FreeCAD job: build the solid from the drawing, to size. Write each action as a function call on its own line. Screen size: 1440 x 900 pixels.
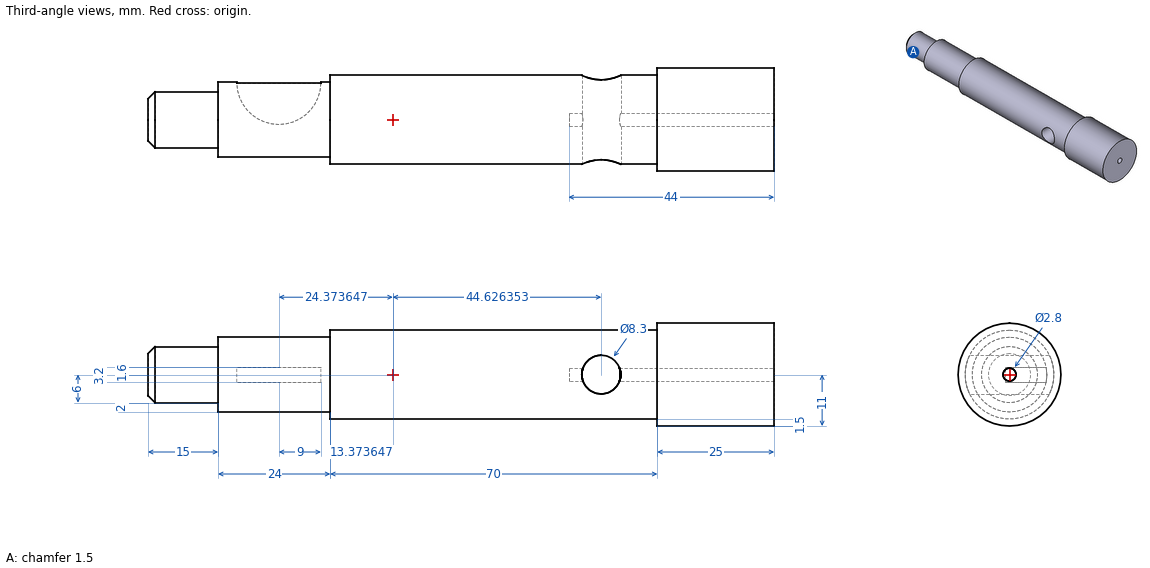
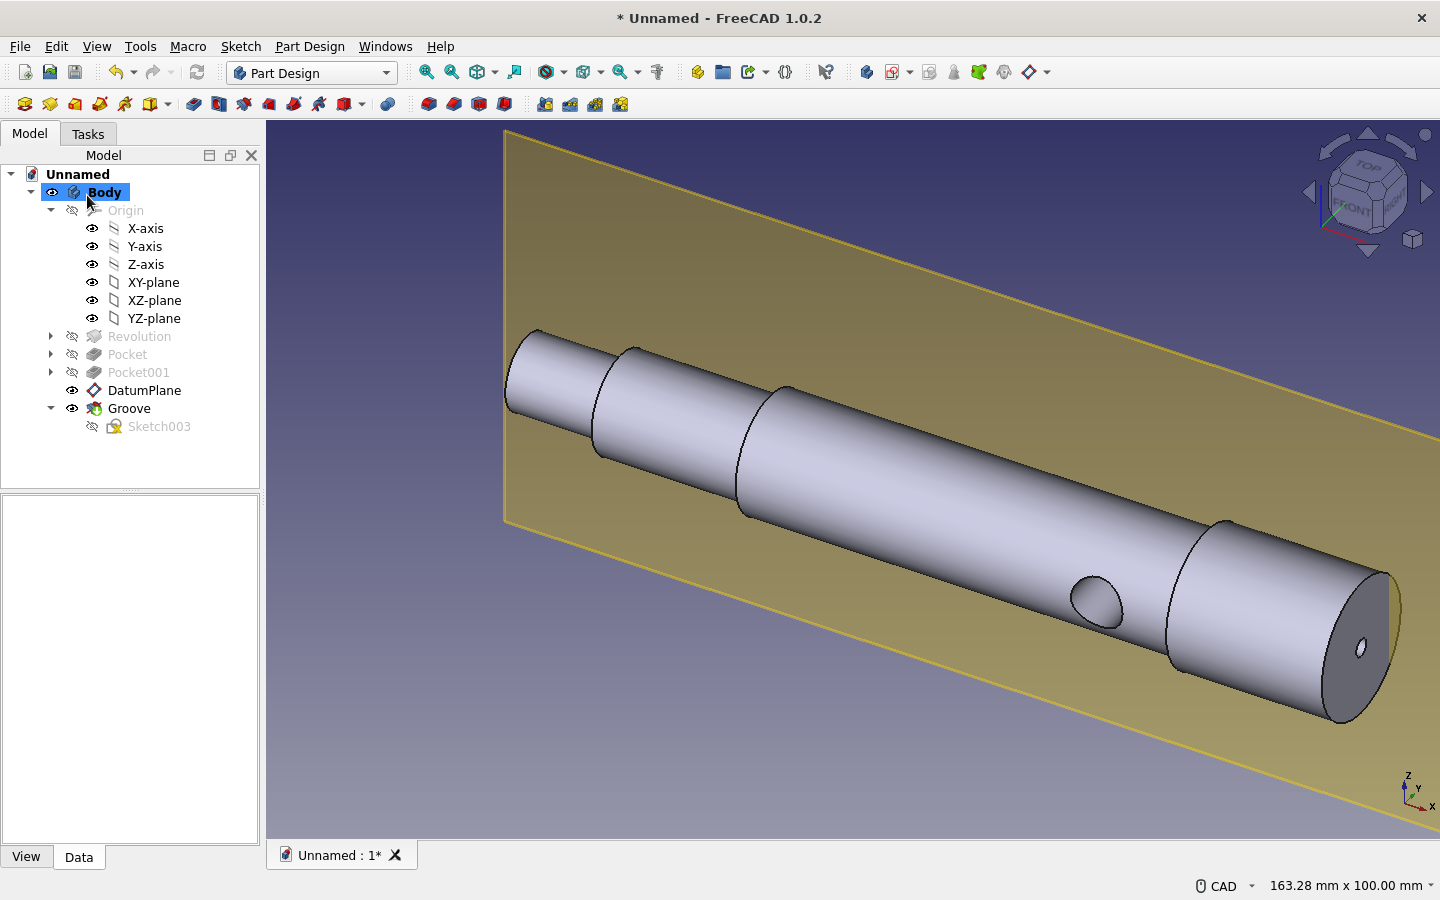
click(117, 390)
key(space)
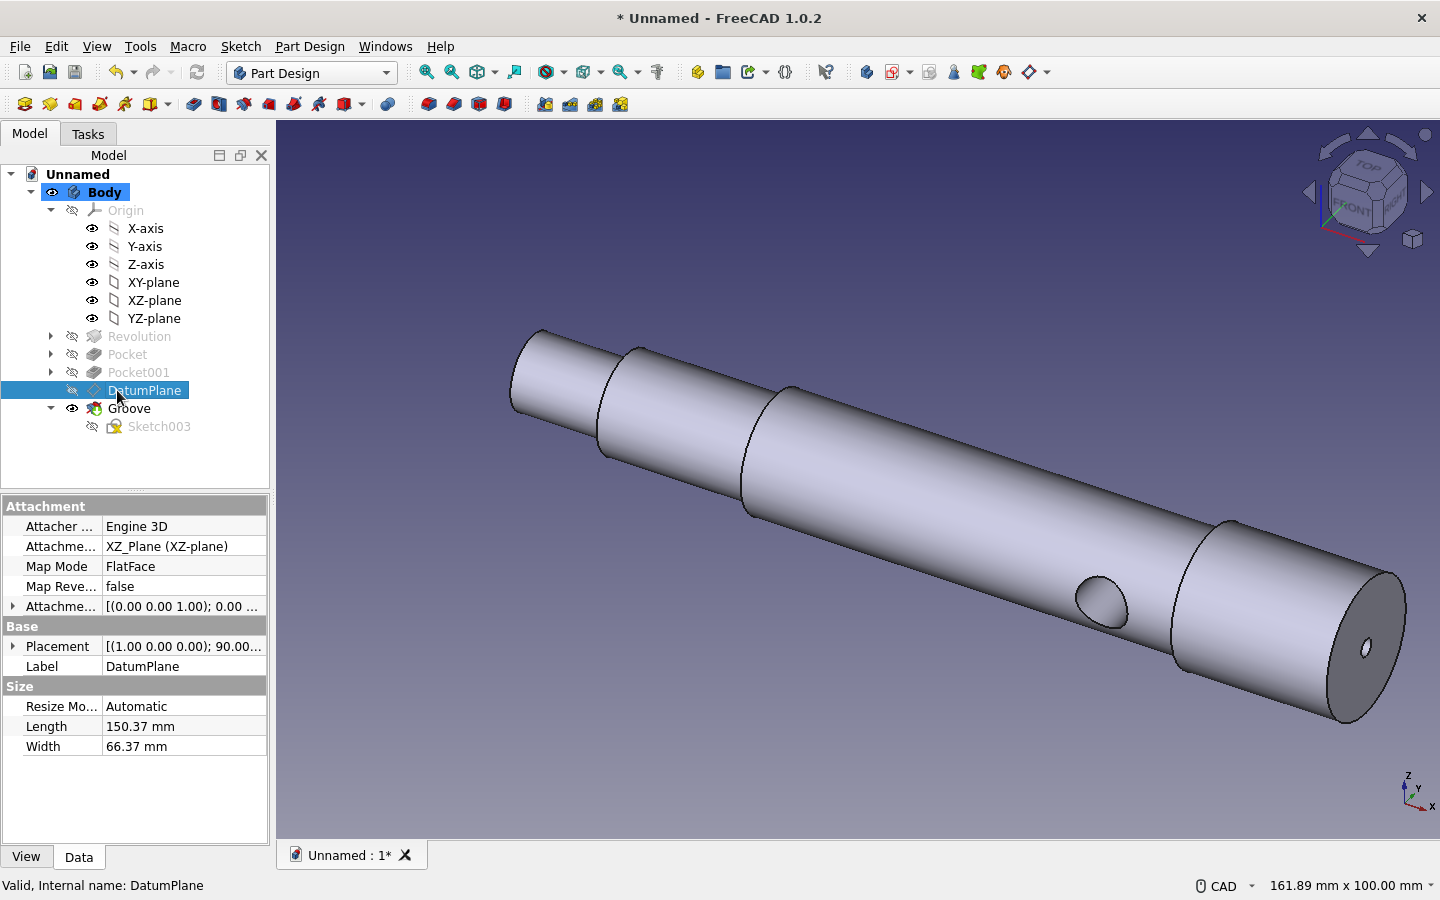
click(519, 355)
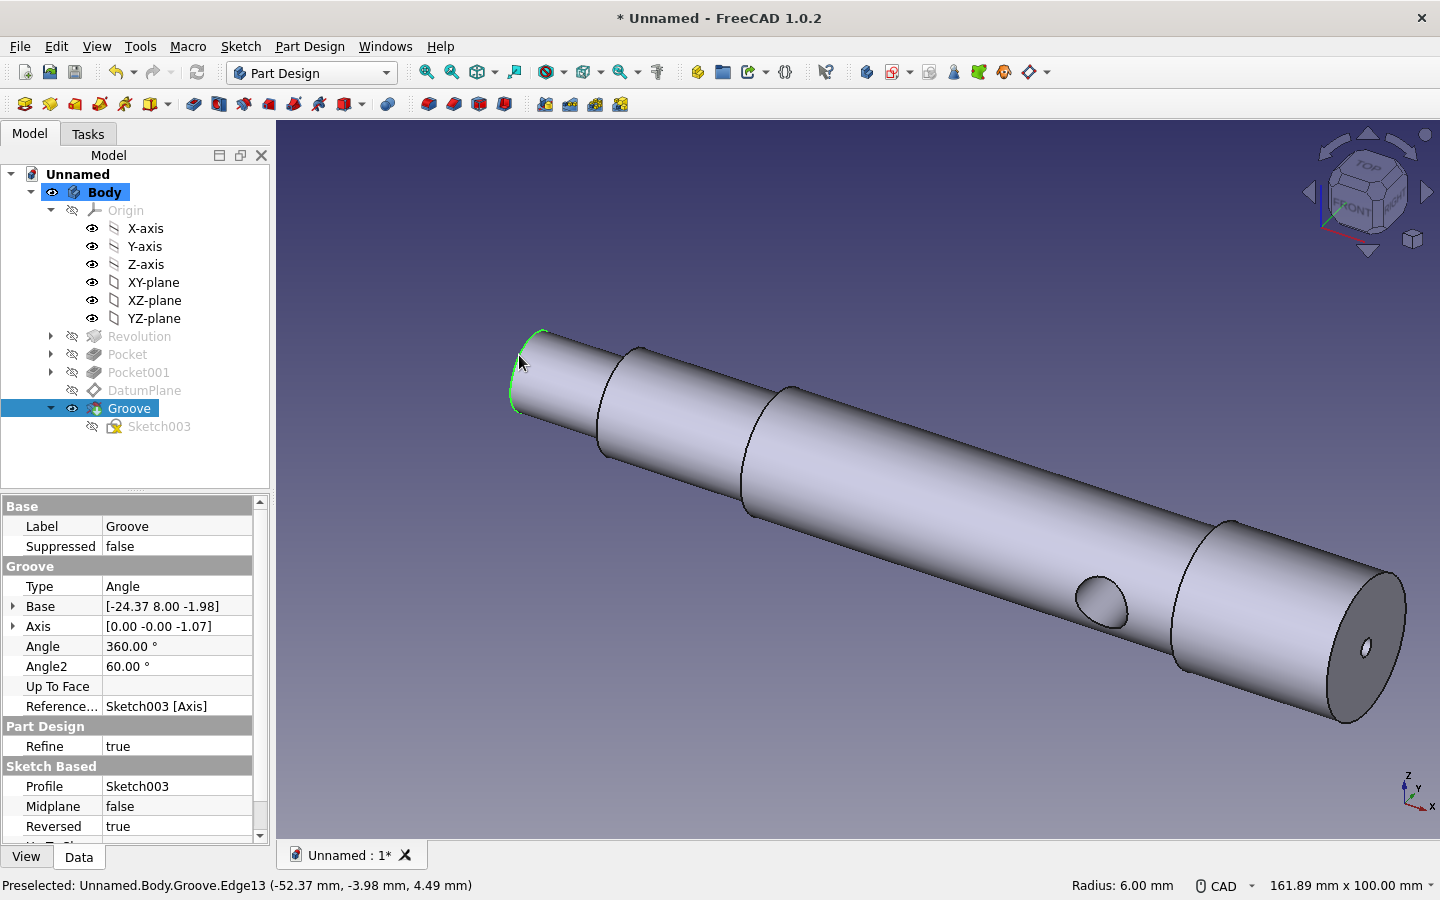
click(454, 104)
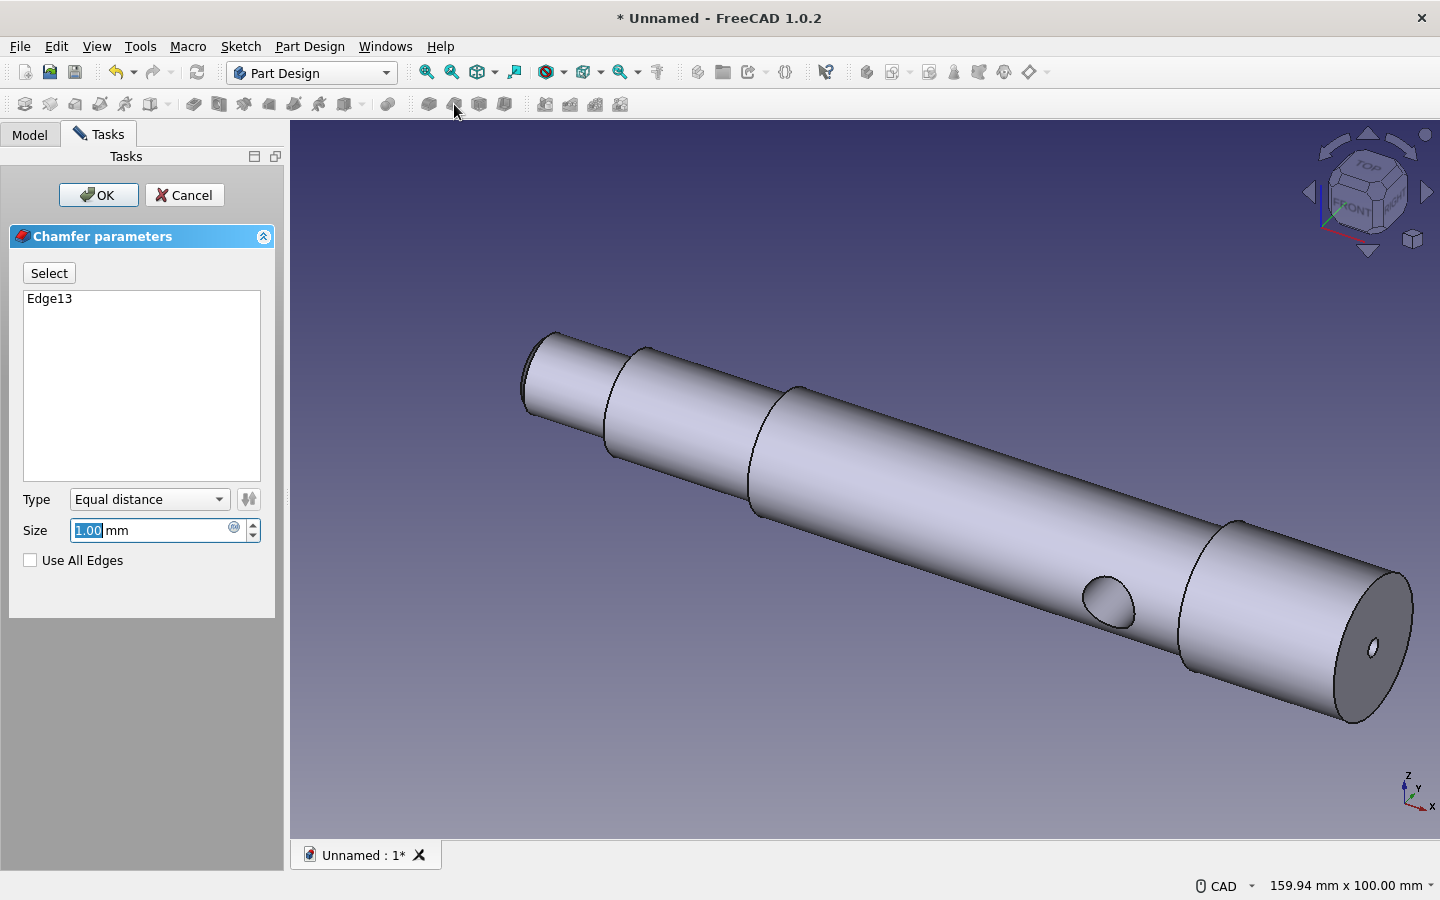
text(1.5)
key(Tab)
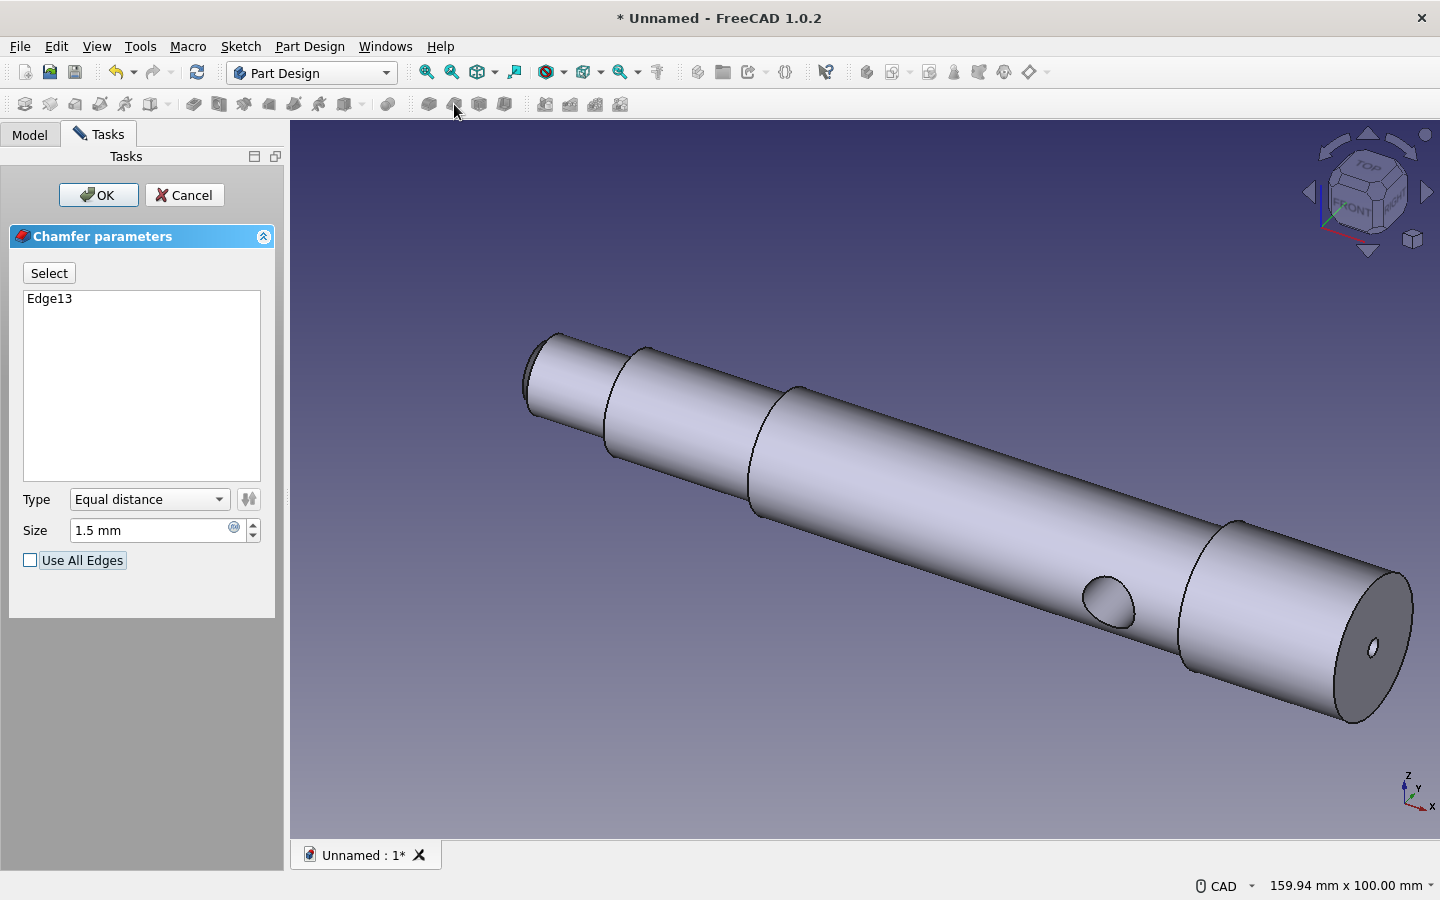
click(99, 195)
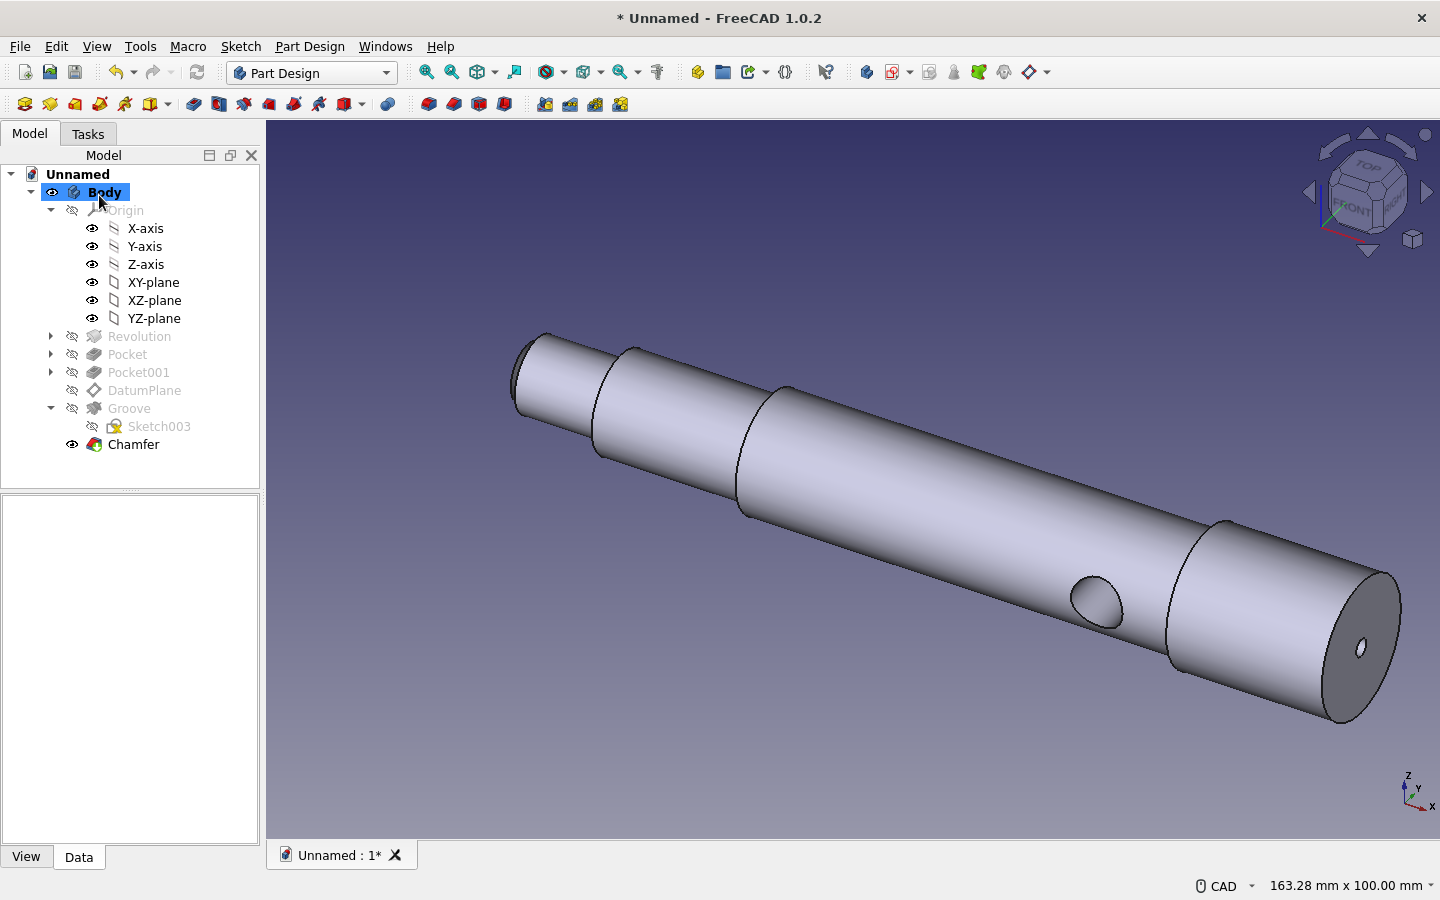
key(0)